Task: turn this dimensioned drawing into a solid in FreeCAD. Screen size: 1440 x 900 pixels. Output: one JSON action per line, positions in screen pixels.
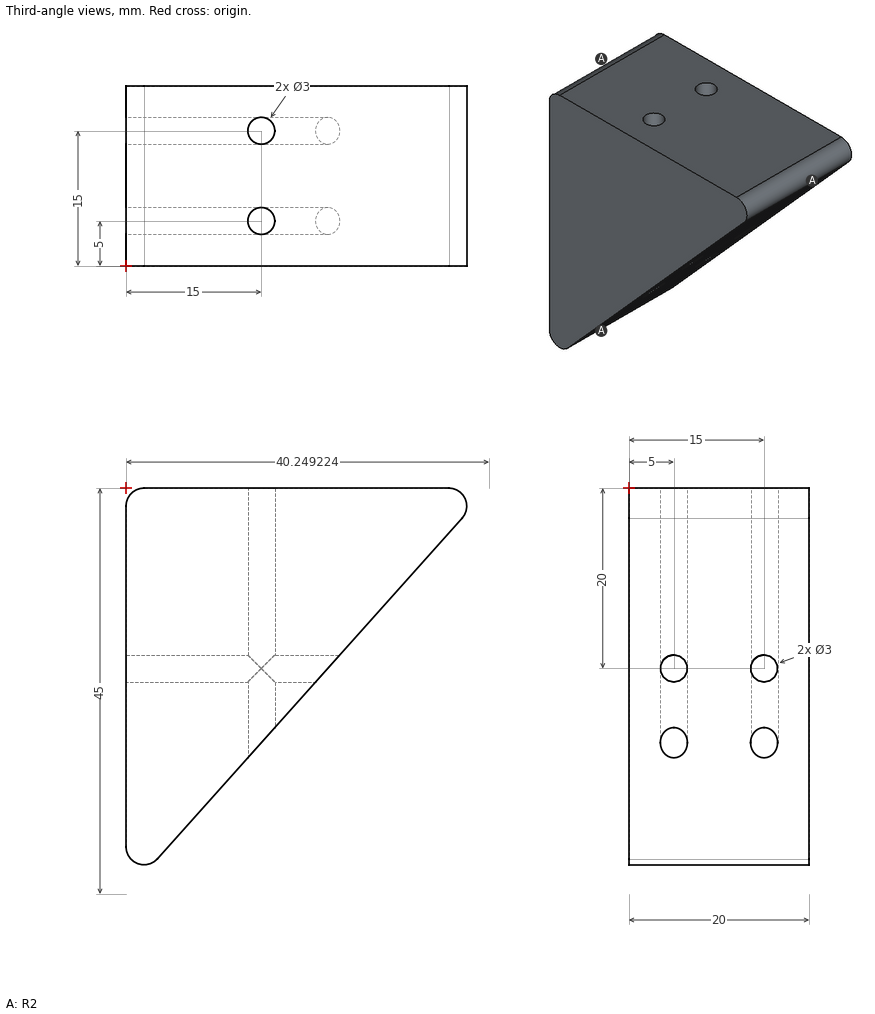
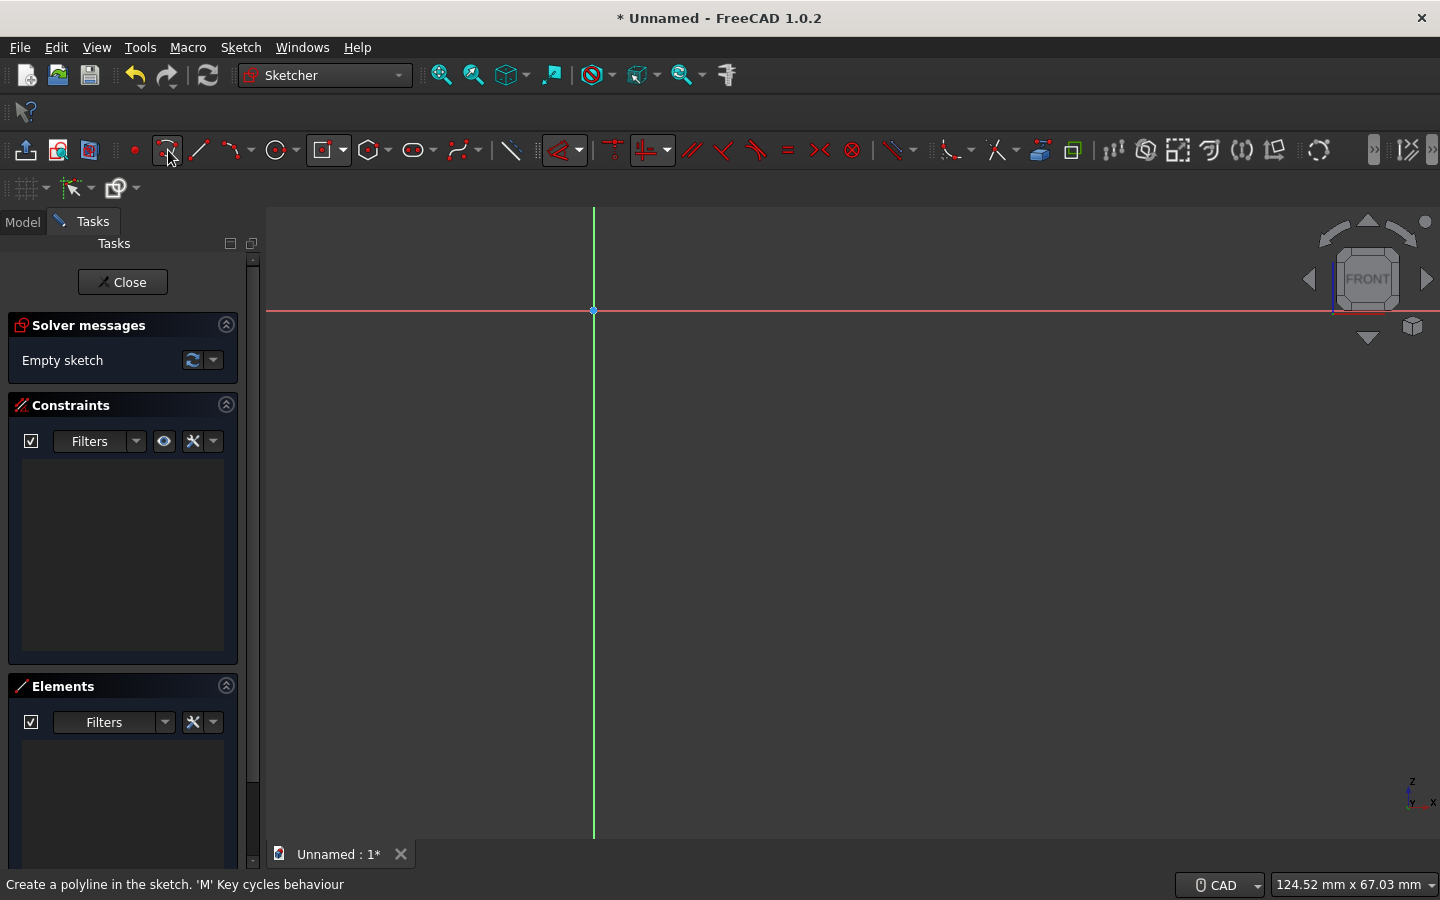
{"action": "left_click", "coordinate": [594, 311]}
{"action": "left_click", "coordinate": [973, 320]}
{"action": "left_click", "coordinate": [603, 735]}
{"action": "left_click", "coordinate": [594, 311]}
{"action": "key", "text": "Escape"}
{"action": "key", "text": "Escape"}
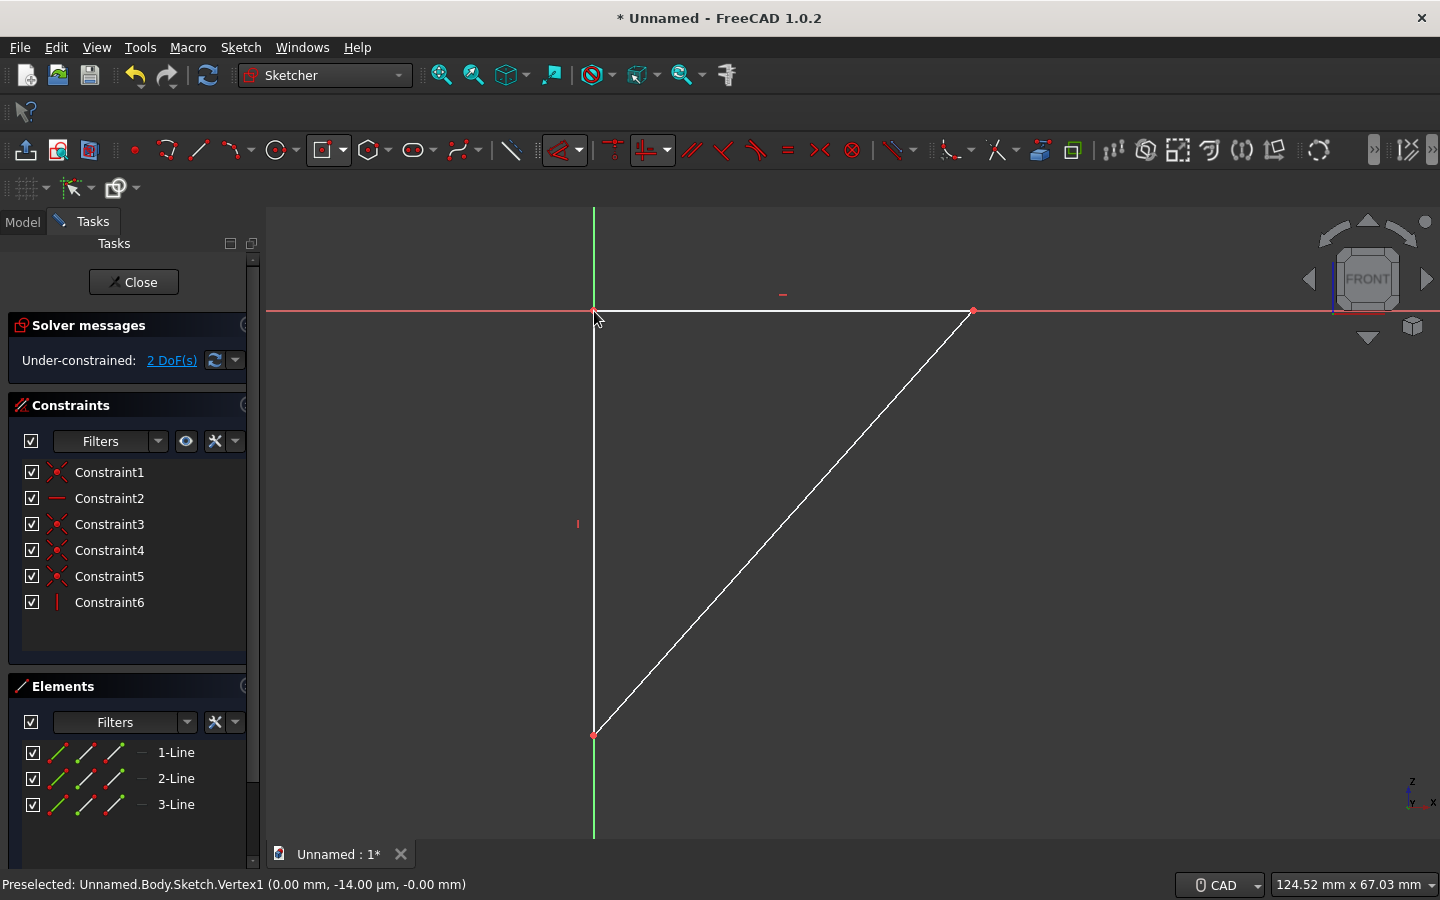
{"action": "key", "text": "d"}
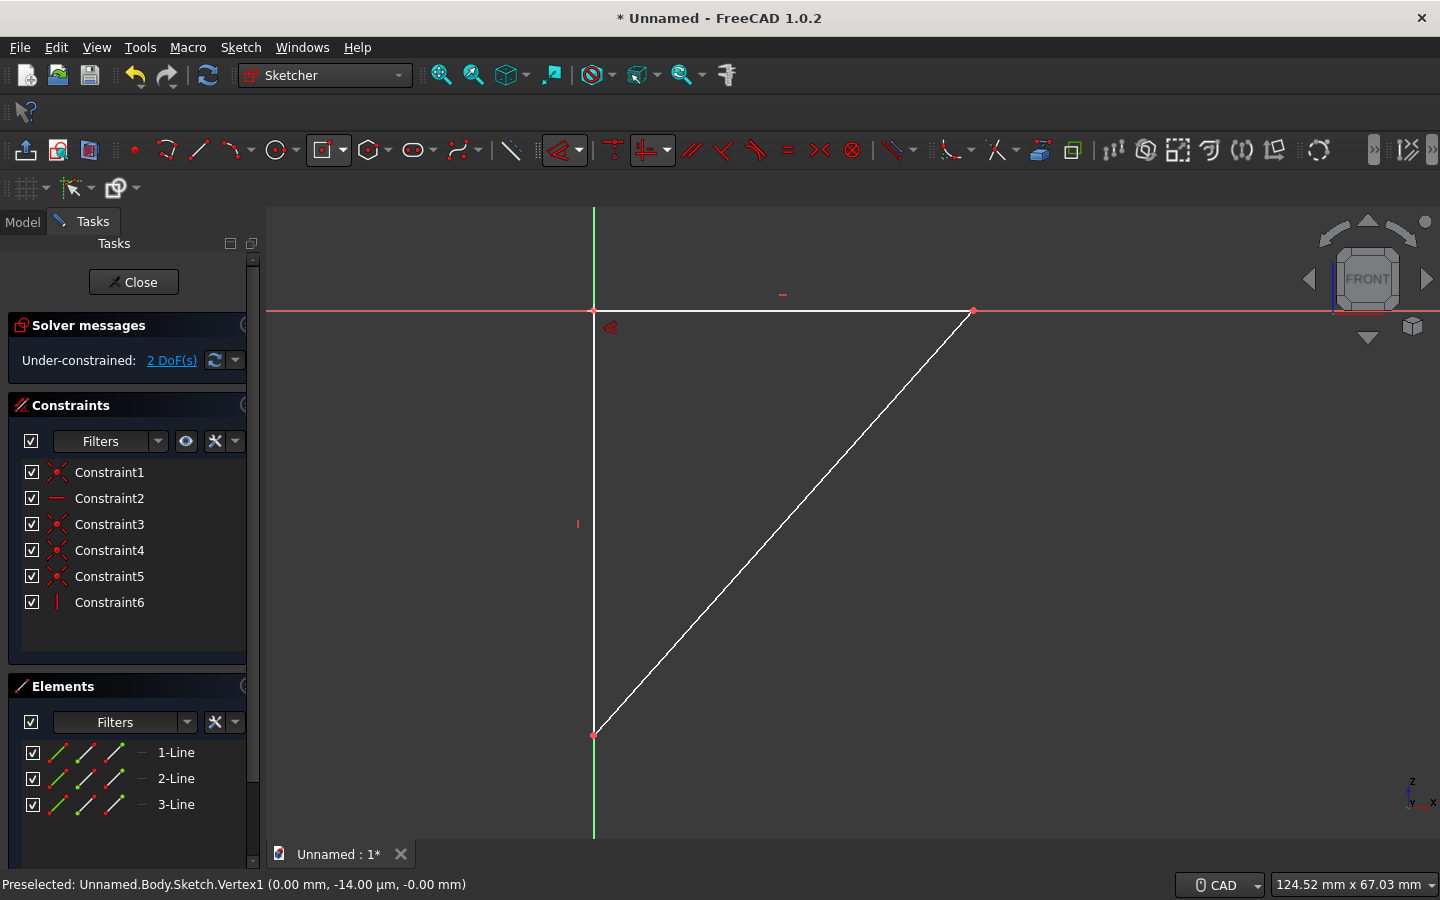
{"action": "left_click", "coordinate": [594, 608]}
{"action": "left_click", "coordinate": [560, 523]}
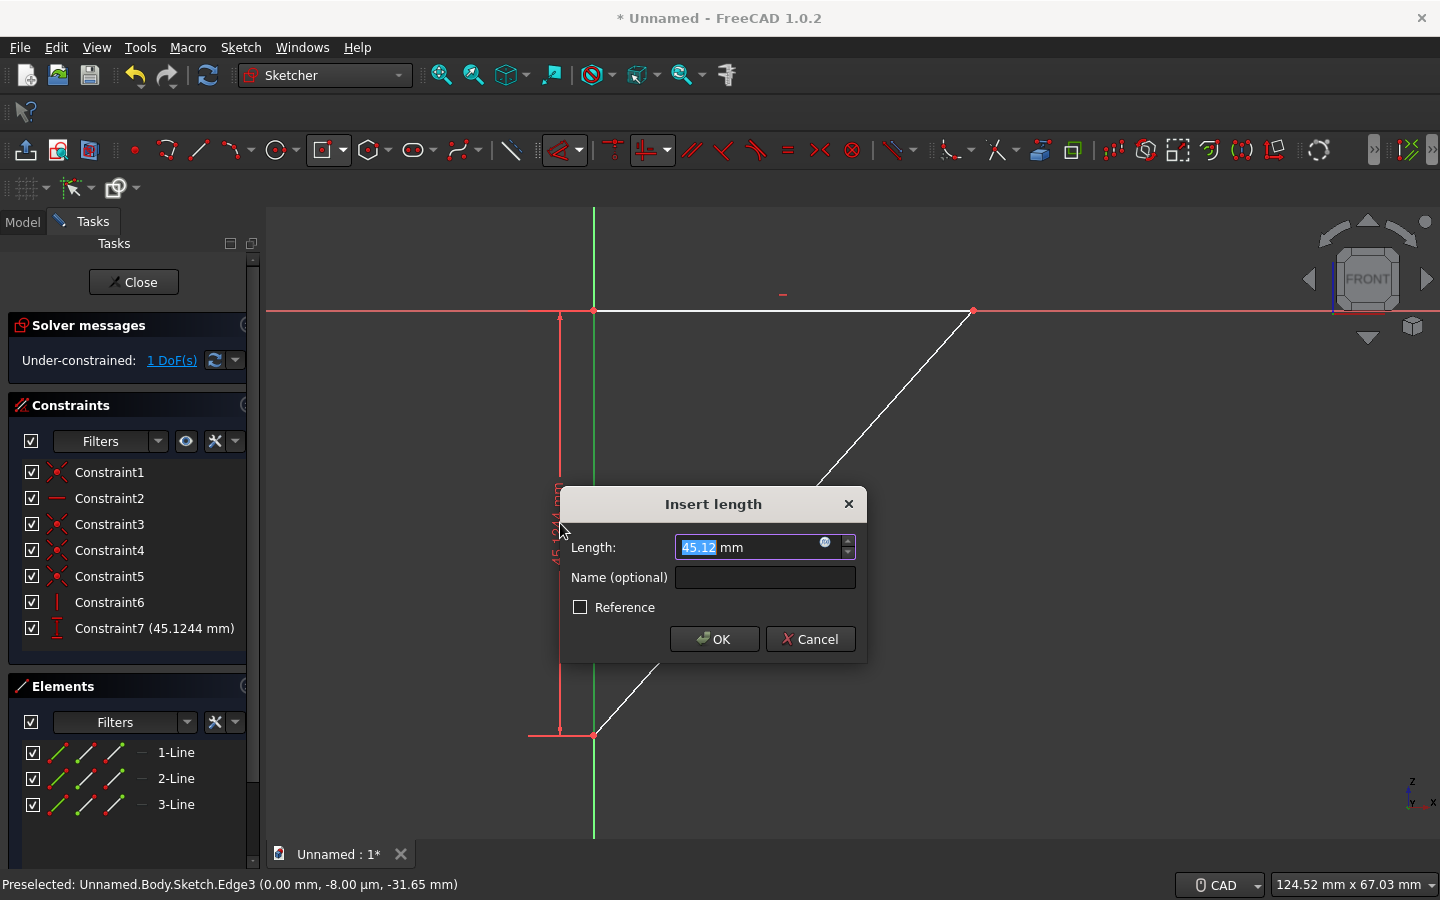
{"action": "type", "text": "45"}
{"action": "key", "text": "Return"}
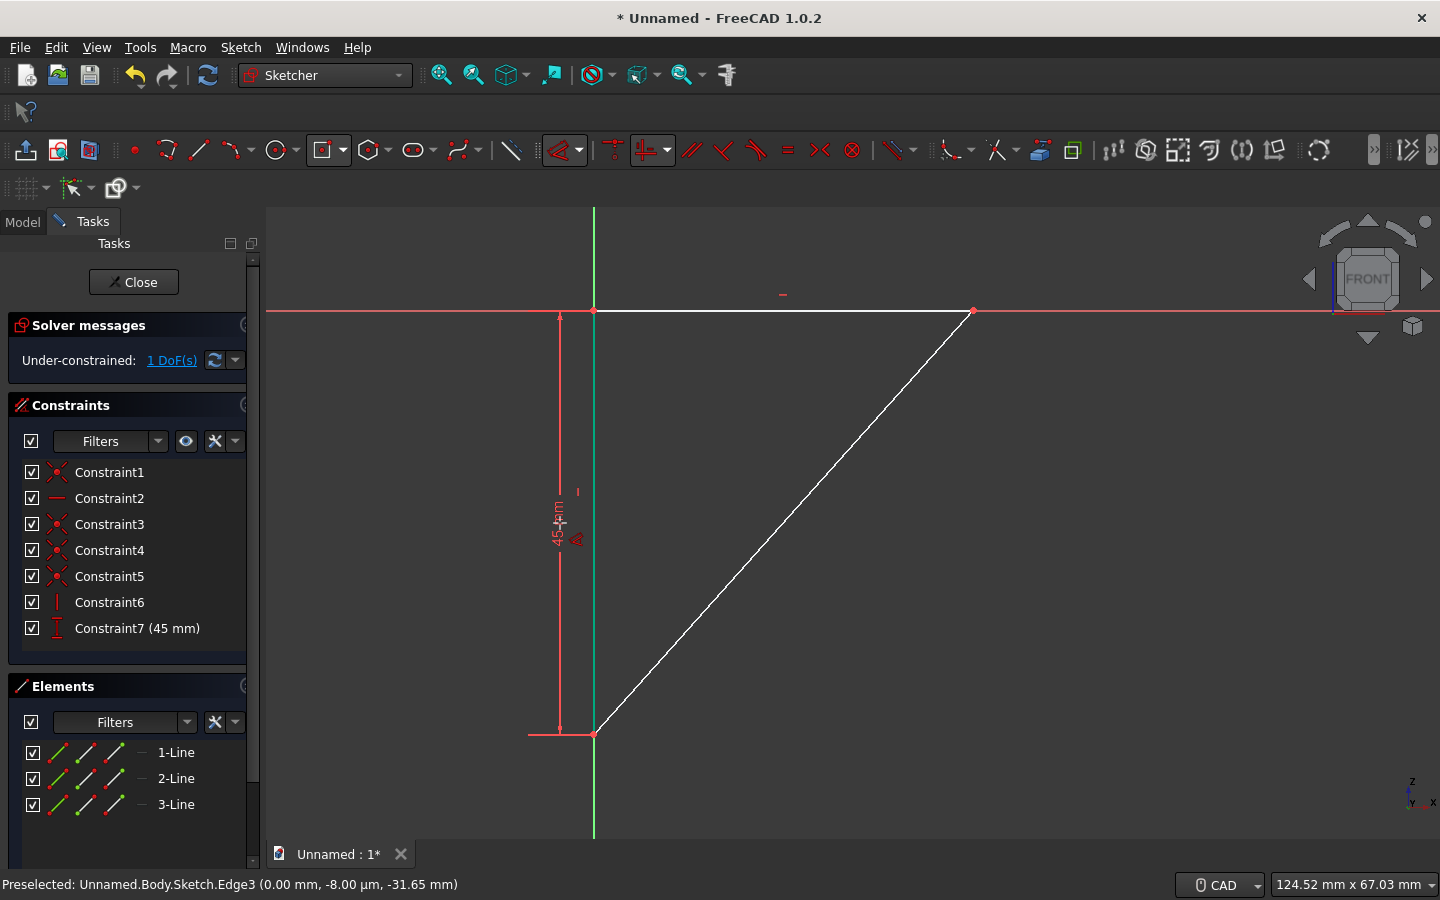
{"action": "left_click", "coordinate": [708, 311]}
{"action": "left_click", "coordinate": [783, 277]}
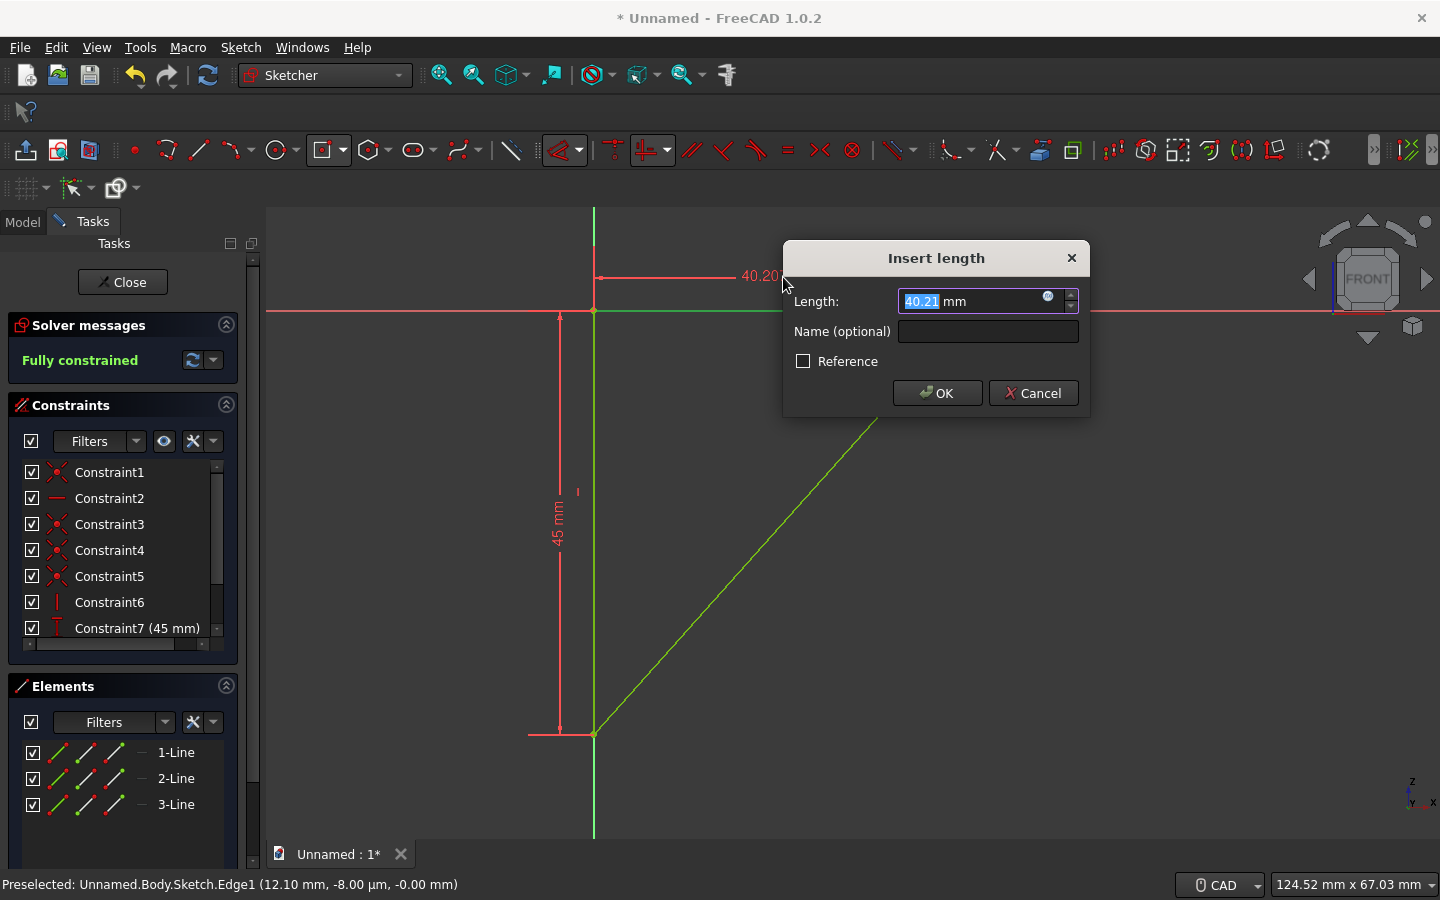
{"action": "type", "text": "40.249224"}
{"action": "key", "text": "Return"}
{"action": "key", "text": "Escape"}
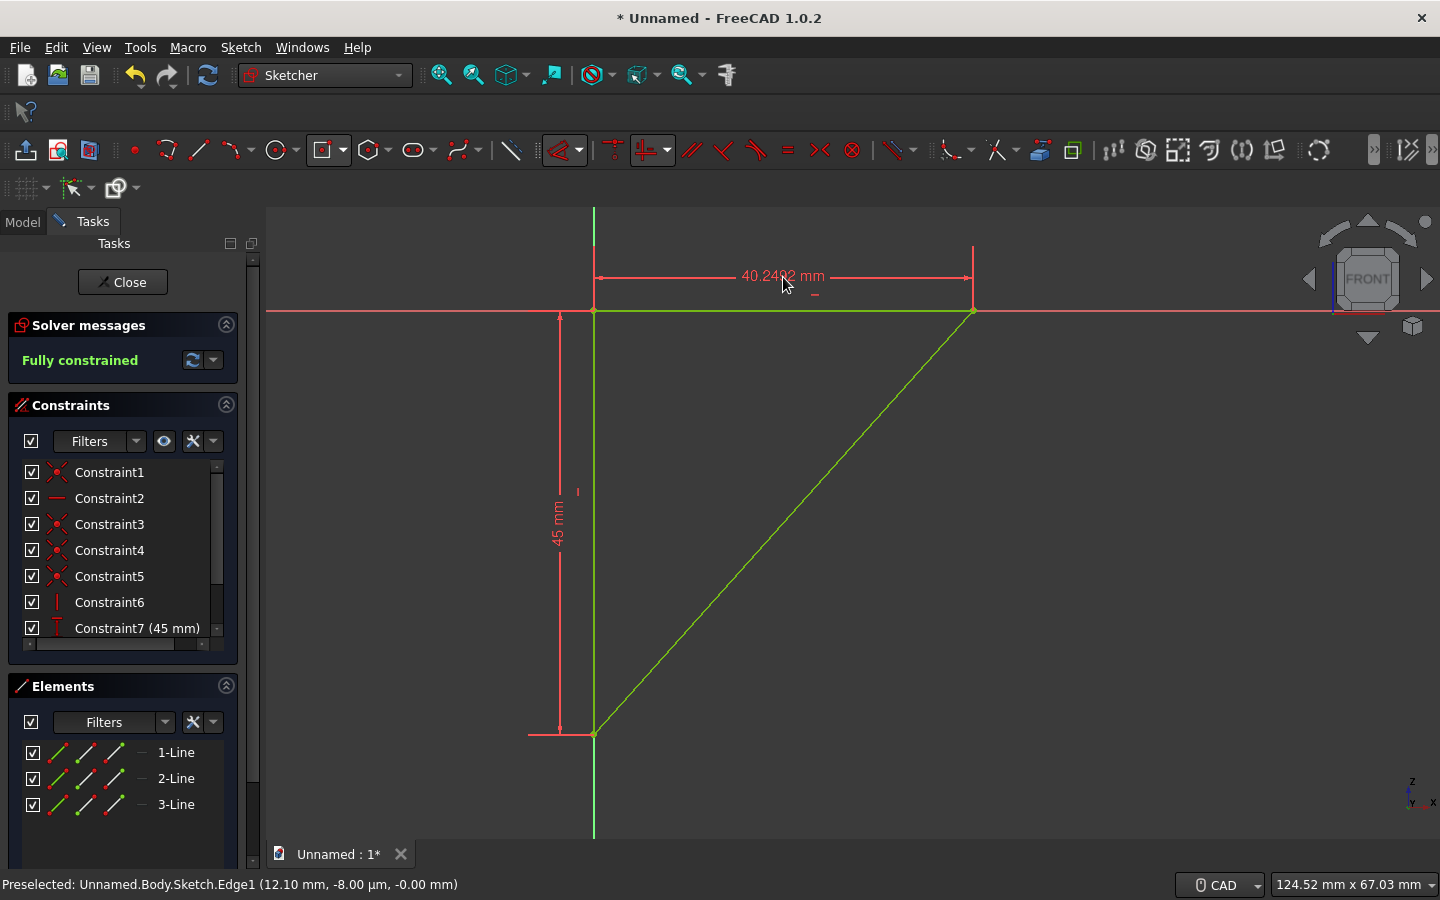
{"action": "left_click", "coordinate": [123, 282]}